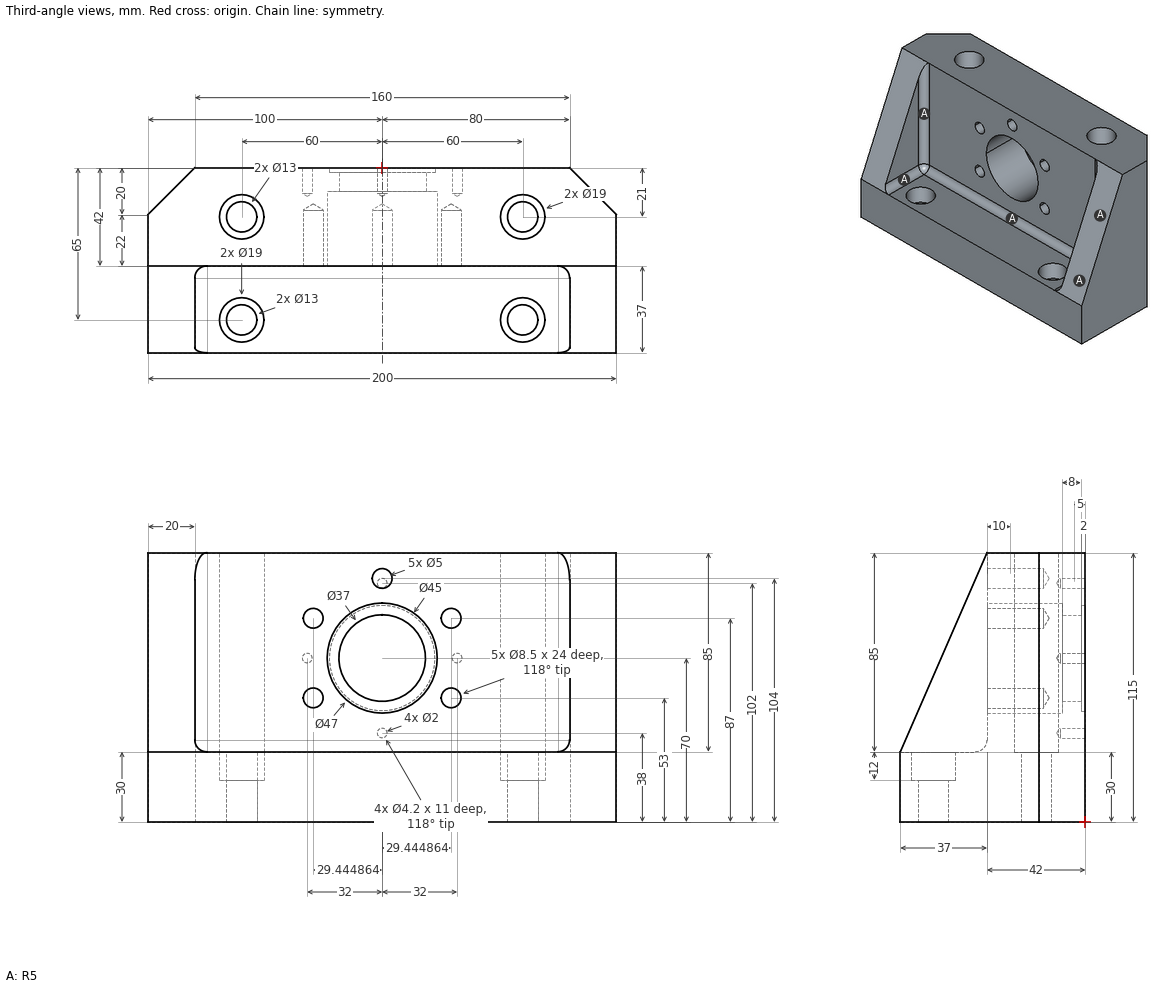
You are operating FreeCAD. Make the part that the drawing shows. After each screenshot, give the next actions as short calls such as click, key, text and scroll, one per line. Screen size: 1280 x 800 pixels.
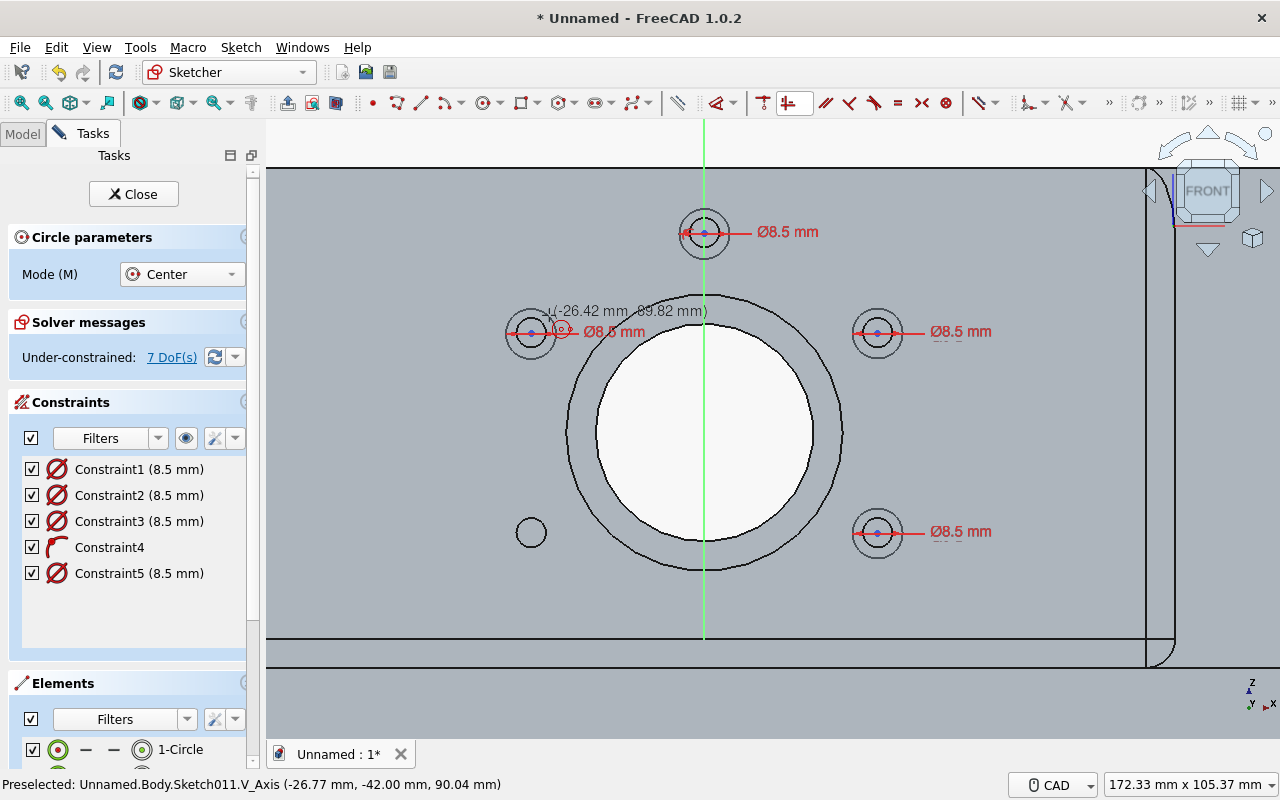
click(531, 533)
move(549, 515)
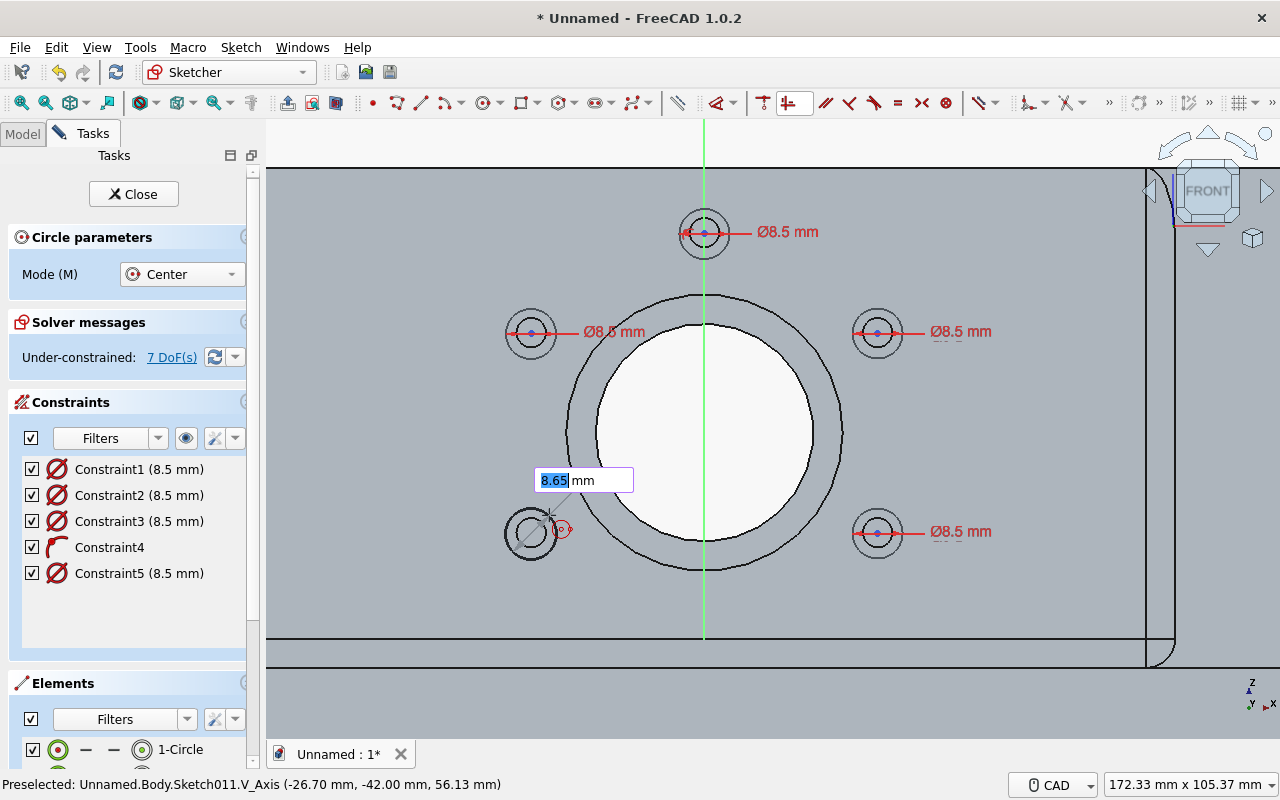
text(8.5)
key(Return)
key(Escape)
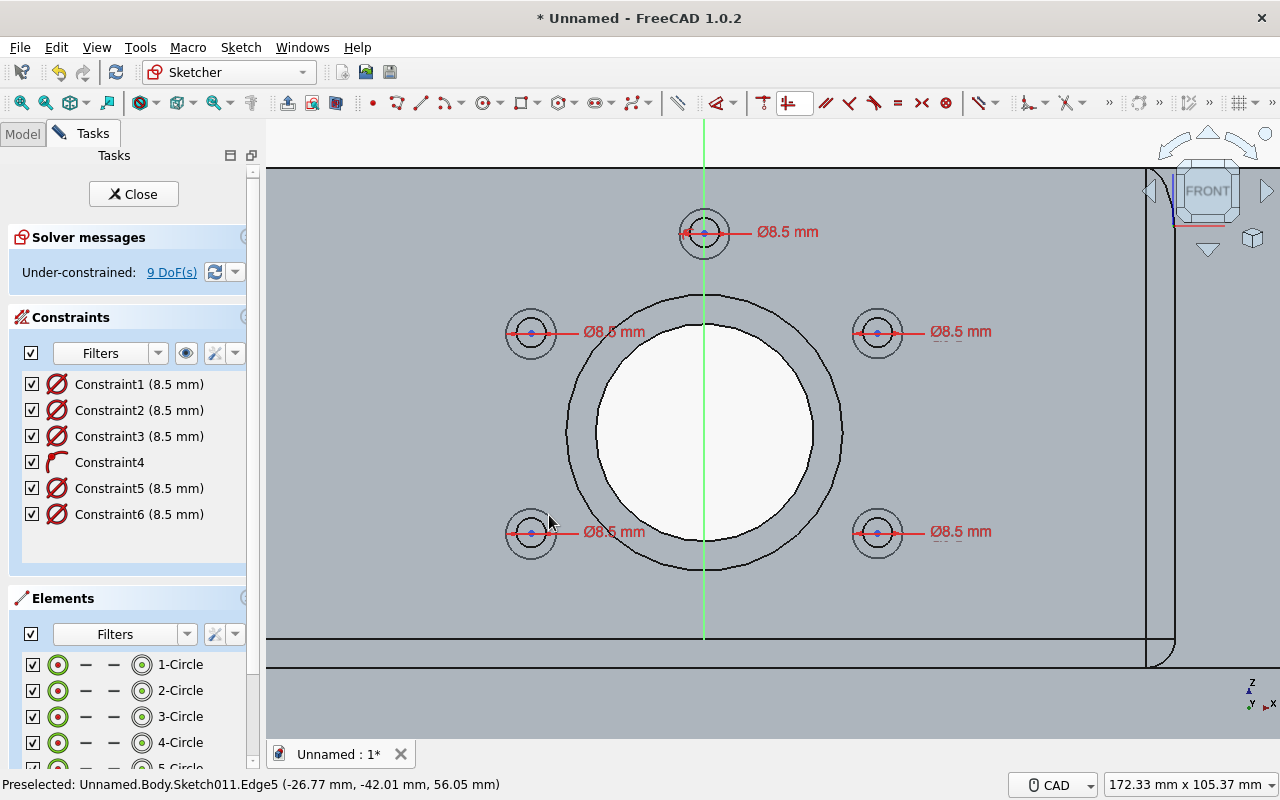
click(878, 534)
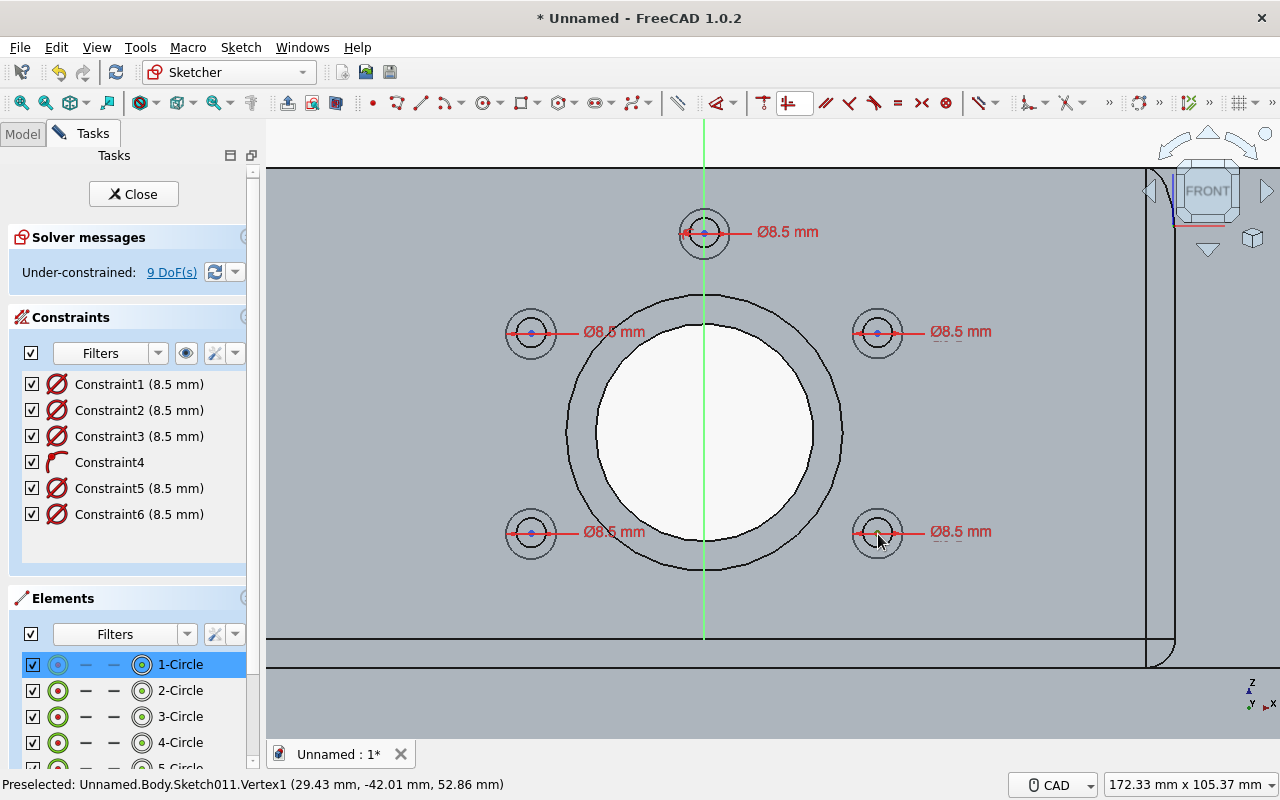
click(878, 334)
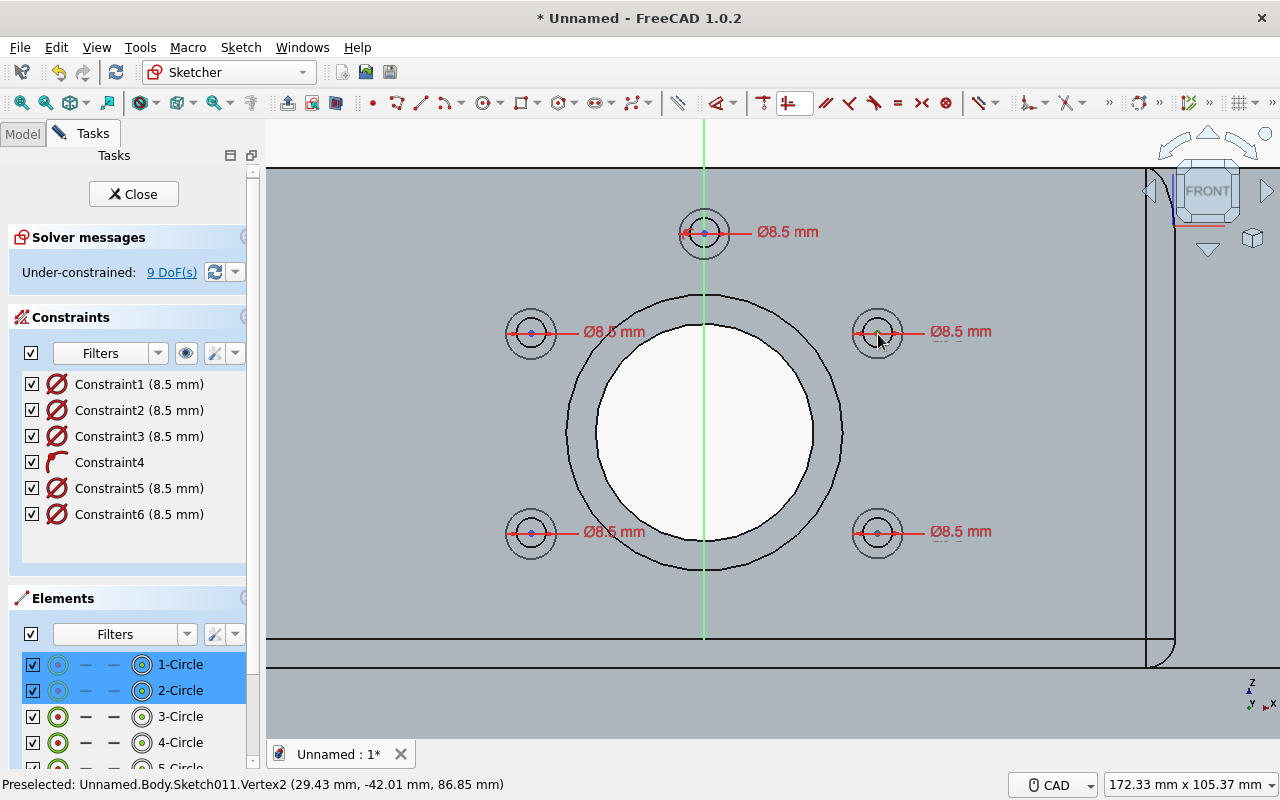
key(v)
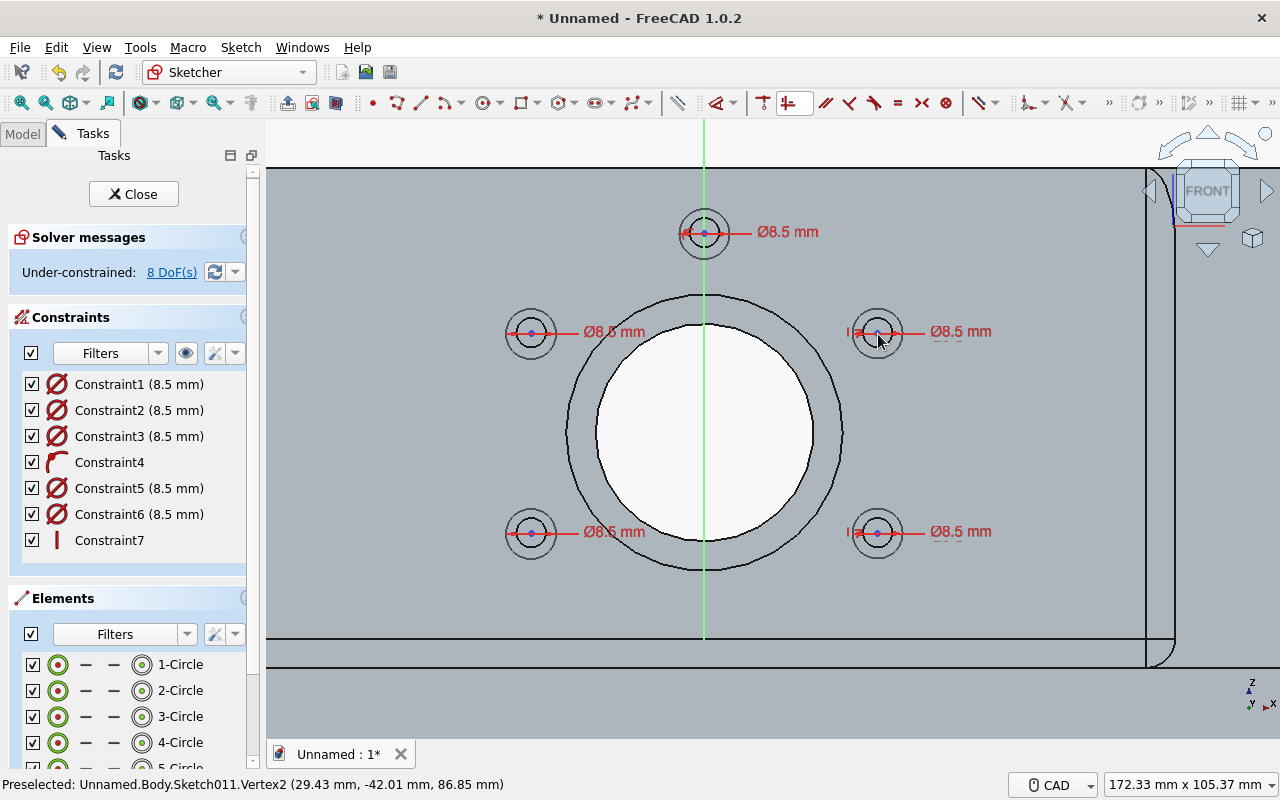
click(878, 334)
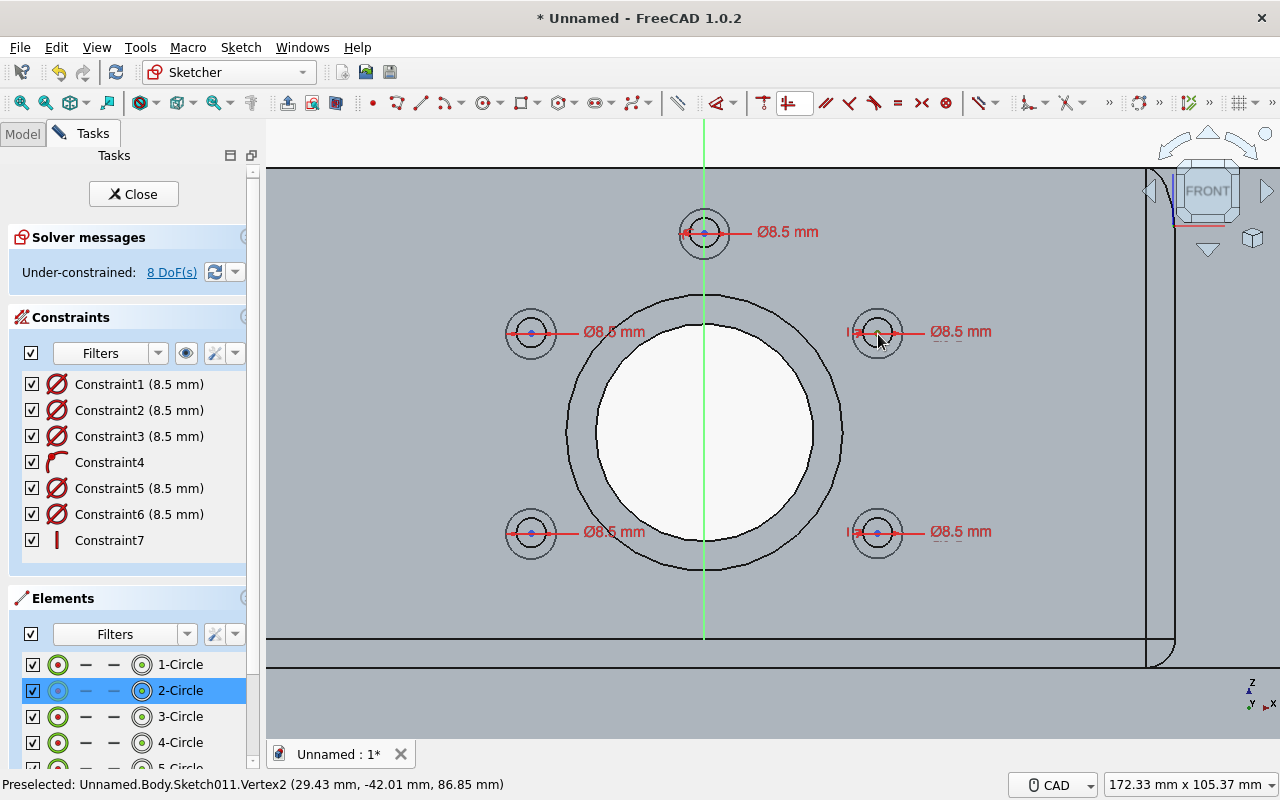
click(531, 334)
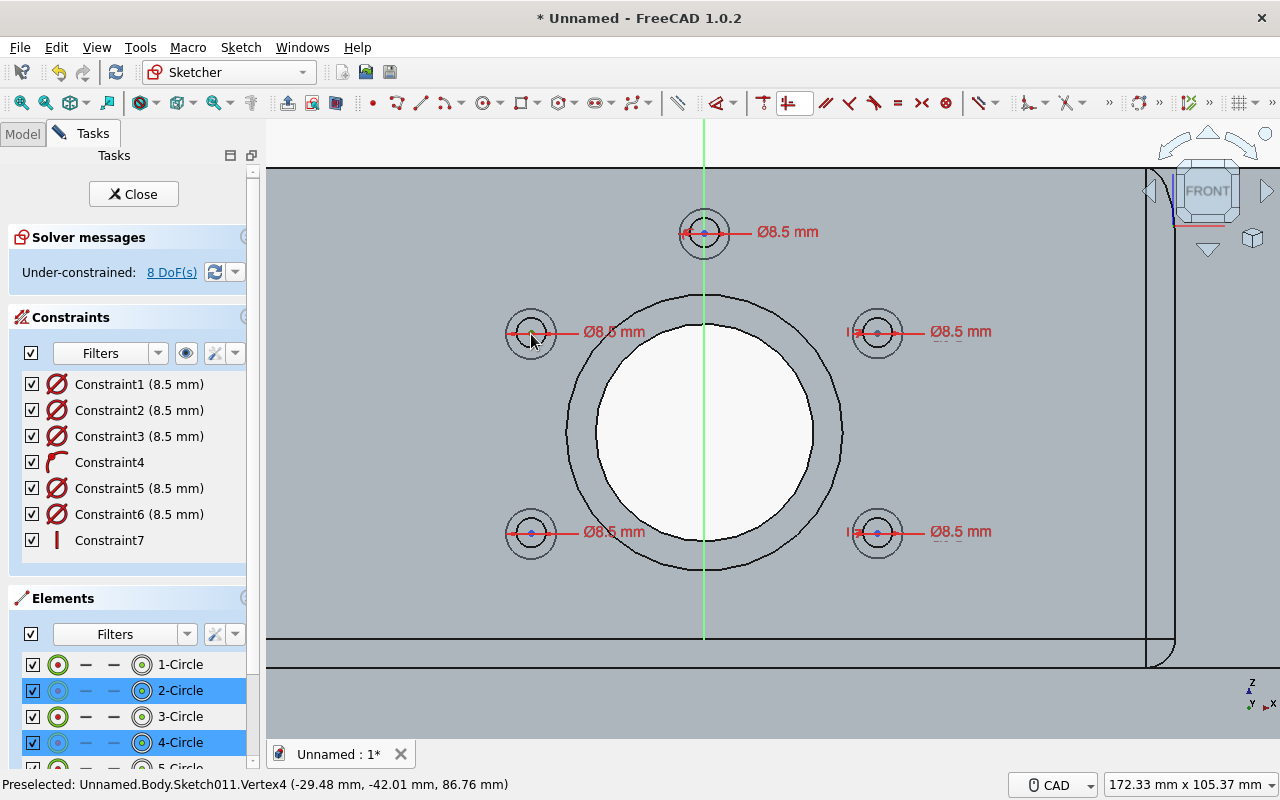
click(808, 104)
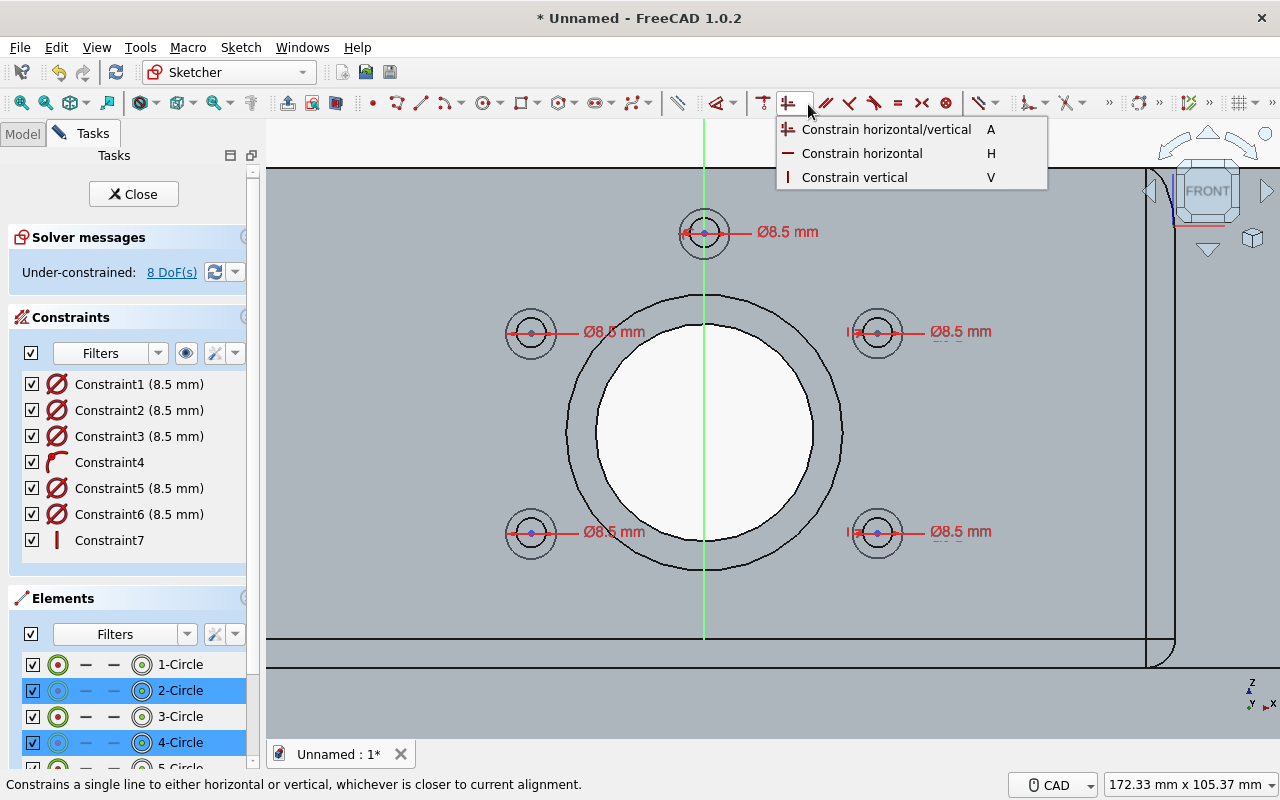
click(912, 153)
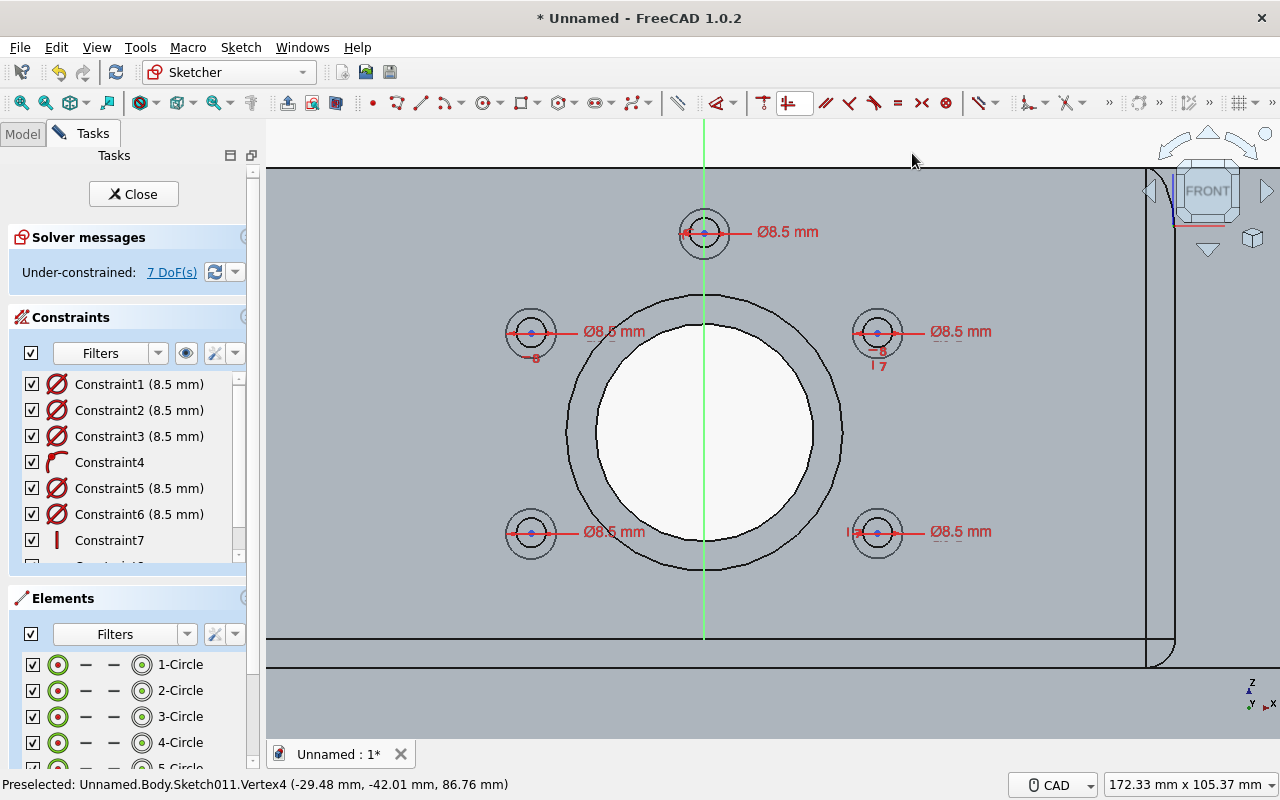
click(531, 334)